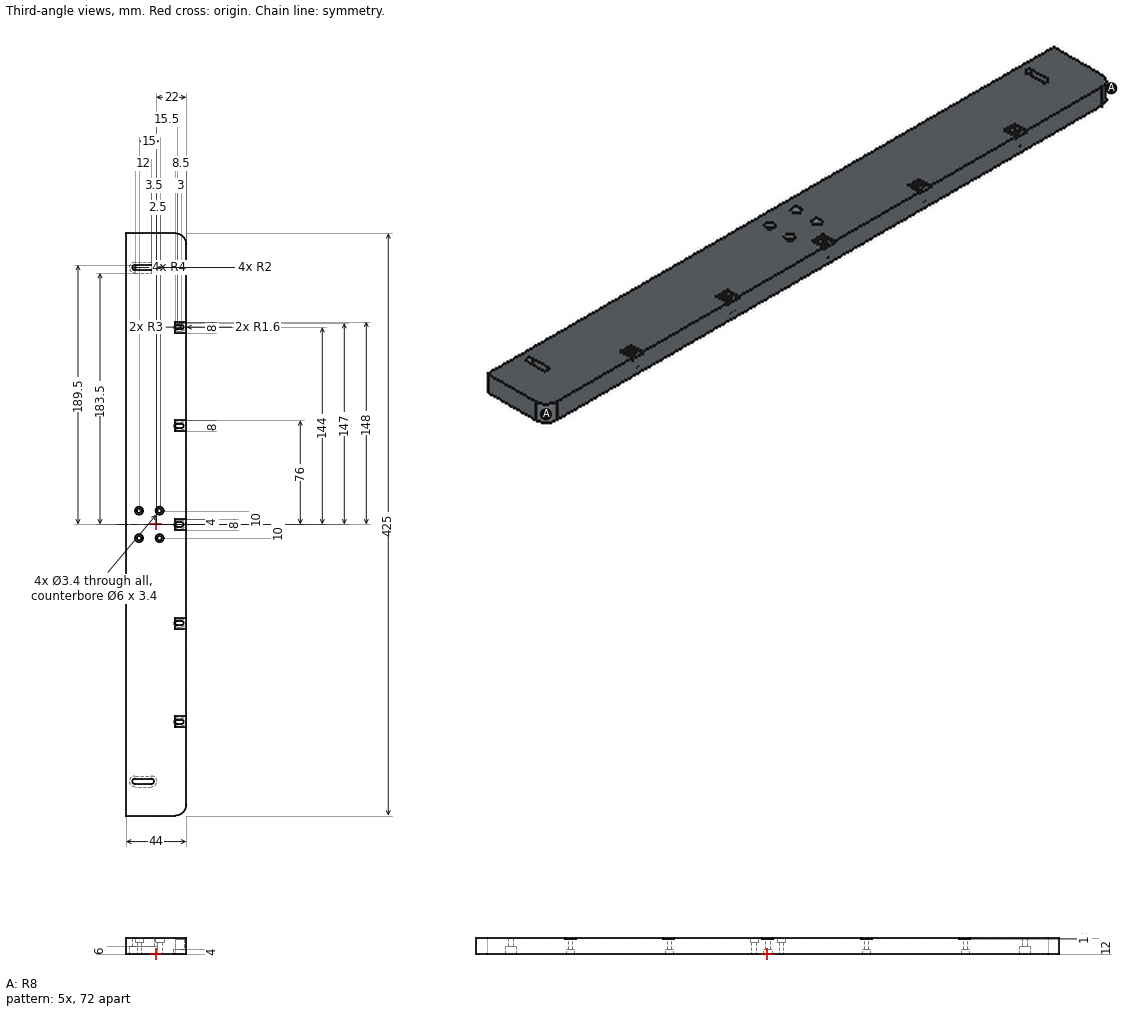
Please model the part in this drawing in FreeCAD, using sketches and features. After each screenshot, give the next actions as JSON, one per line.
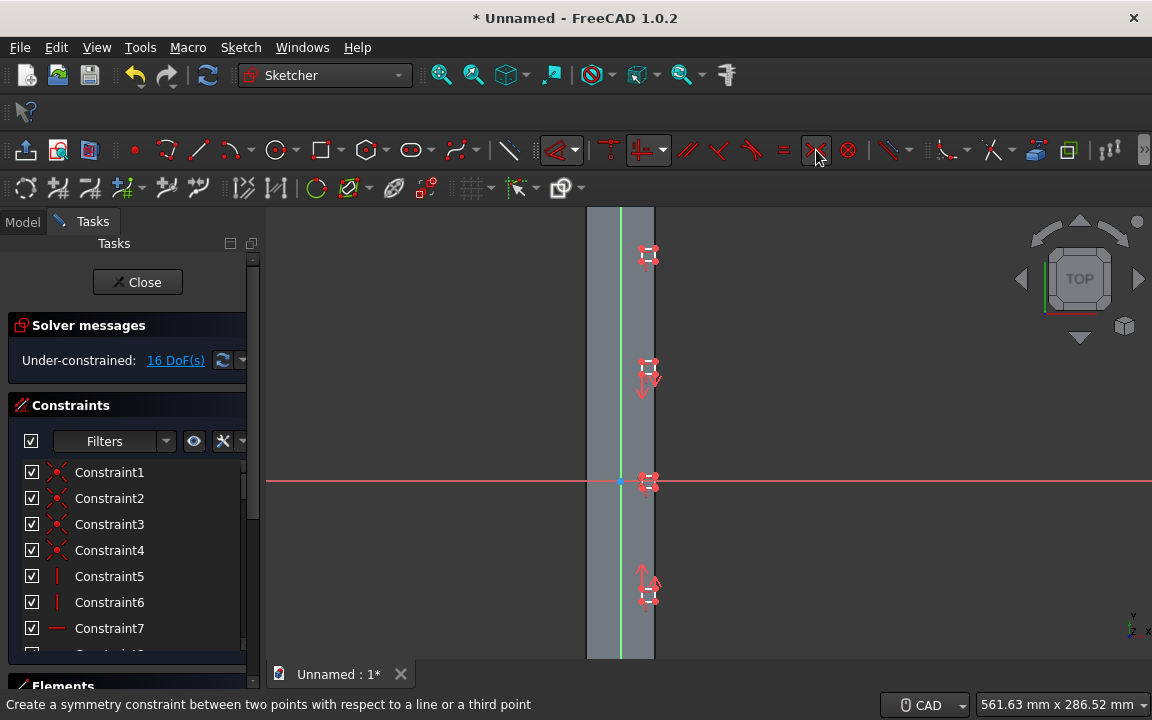
{"action": "left_click", "coordinate": [642, 261]}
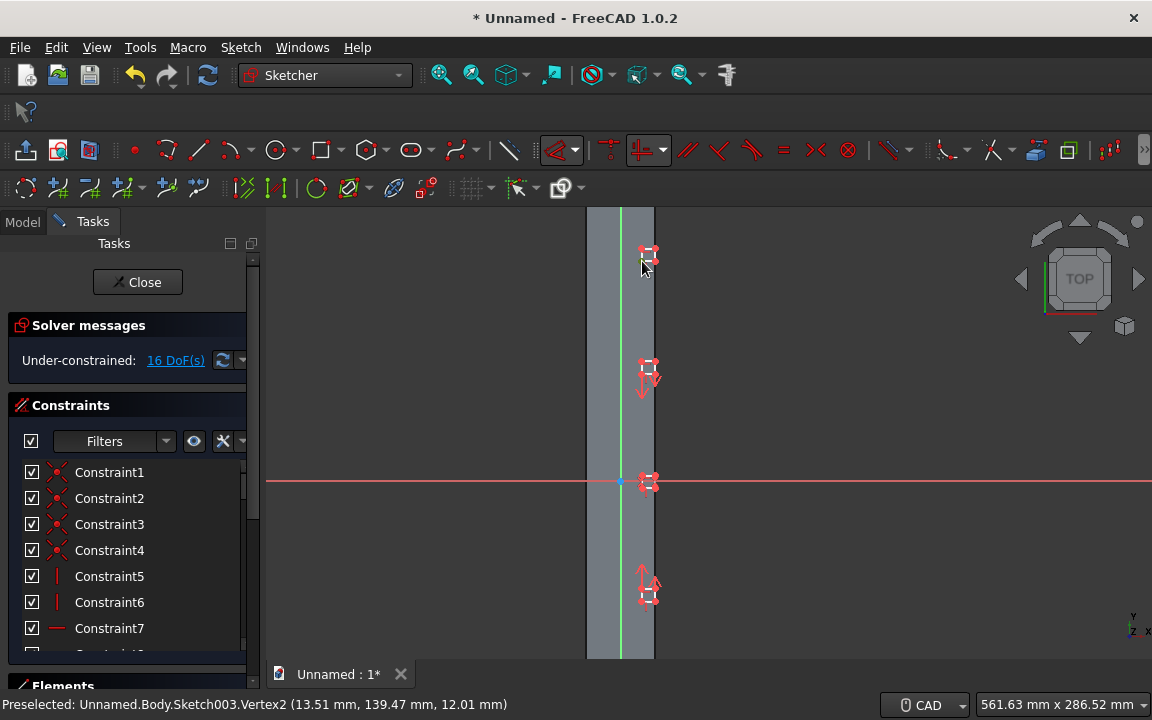
{"action": "scroll", "coordinate": [644, 374], "scroll_direction": "down", "scroll_amount": 3}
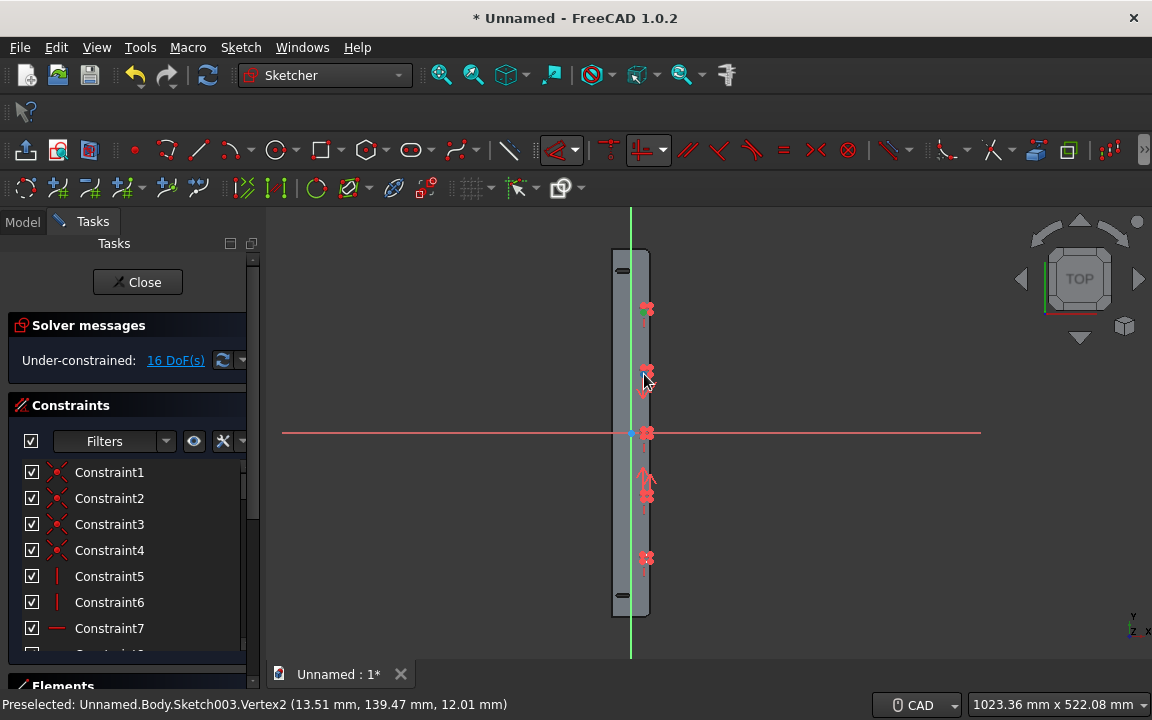
{"action": "scroll", "coordinate": [643, 555], "scroll_direction": "up", "scroll_amount": 3}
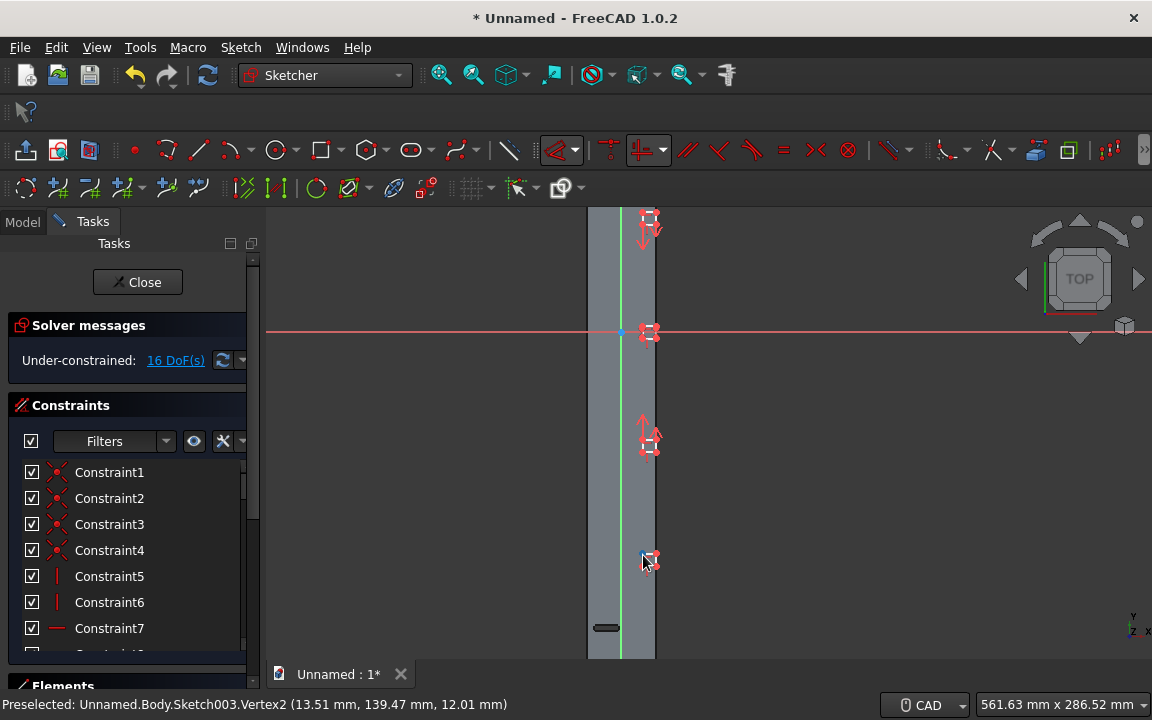
{"action": "left_click", "coordinate": [643, 554]}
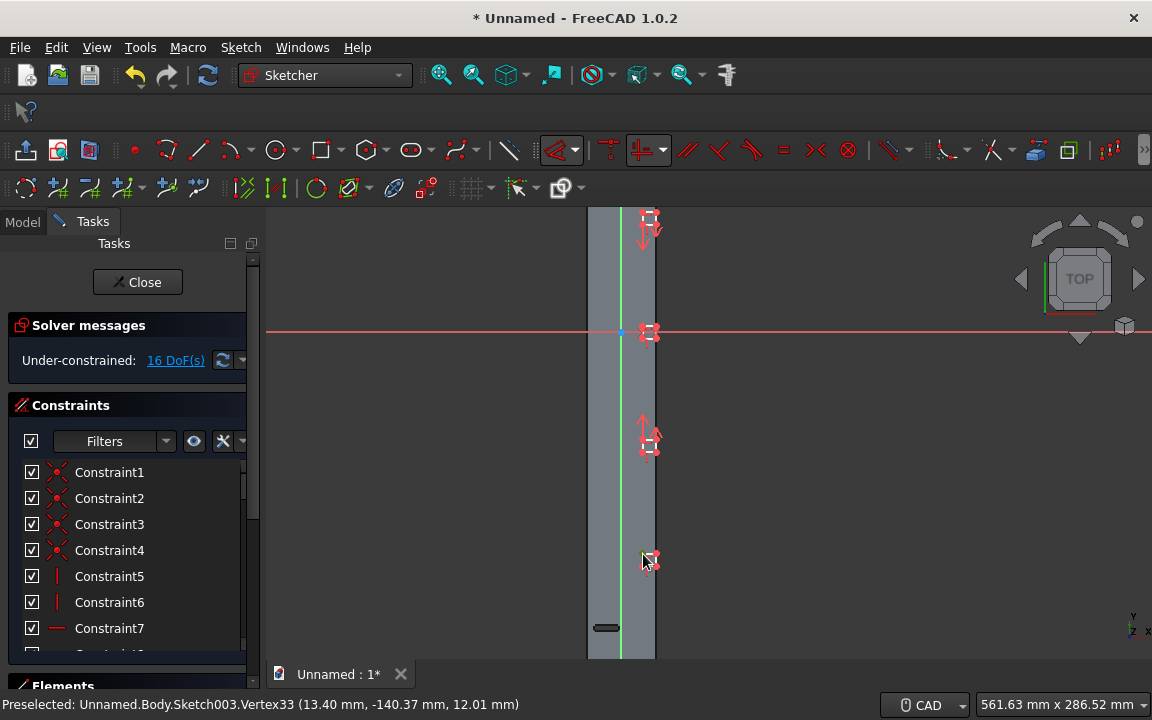
{"action": "left_click", "coordinate": [344, 332]}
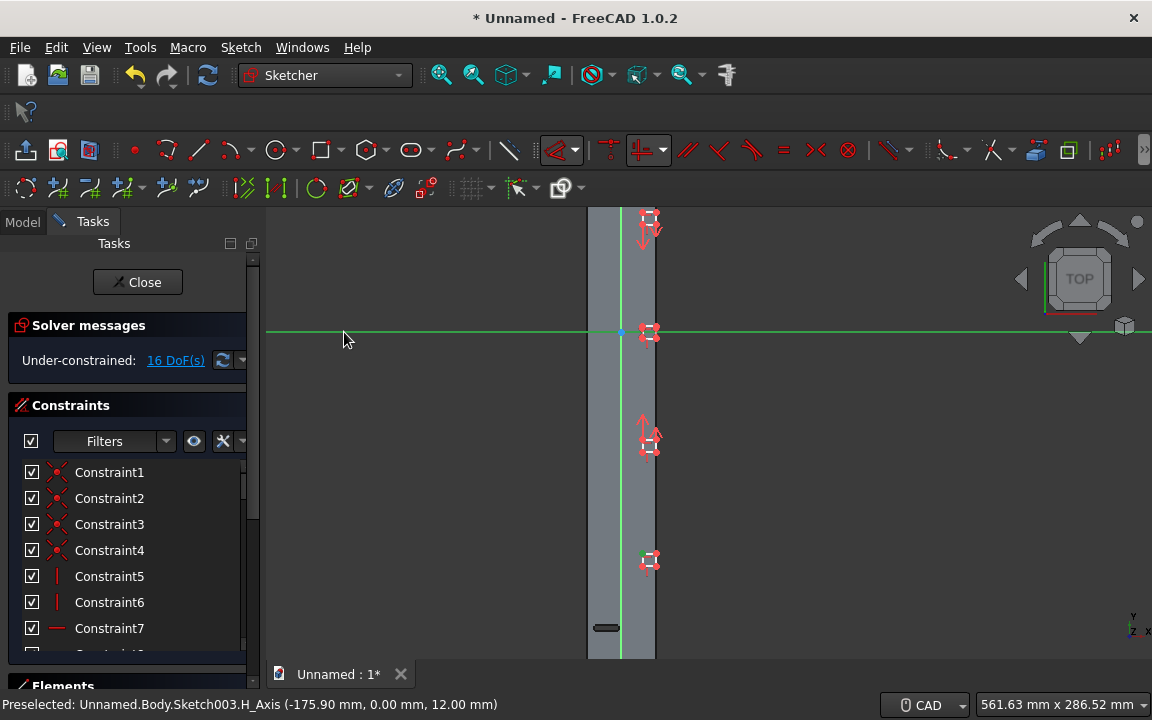
{"action": "key", "text": "s"}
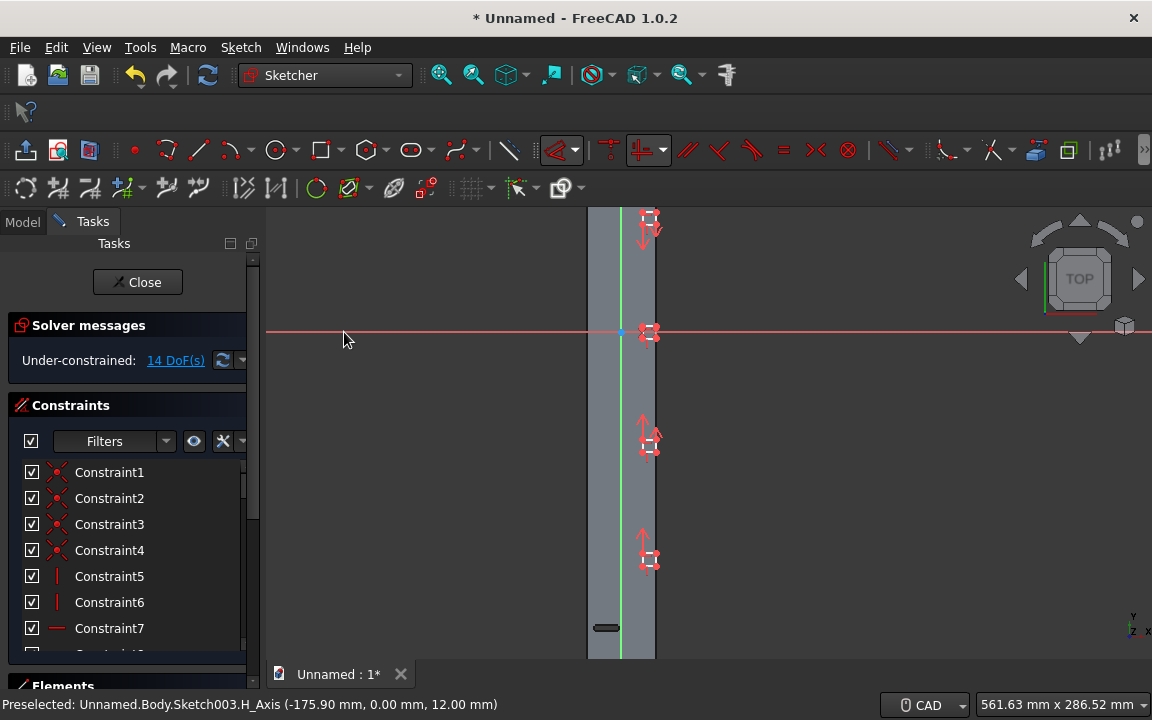
{"action": "scroll", "coordinate": [643, 555], "scroll_direction": "down", "scroll_amount": 3}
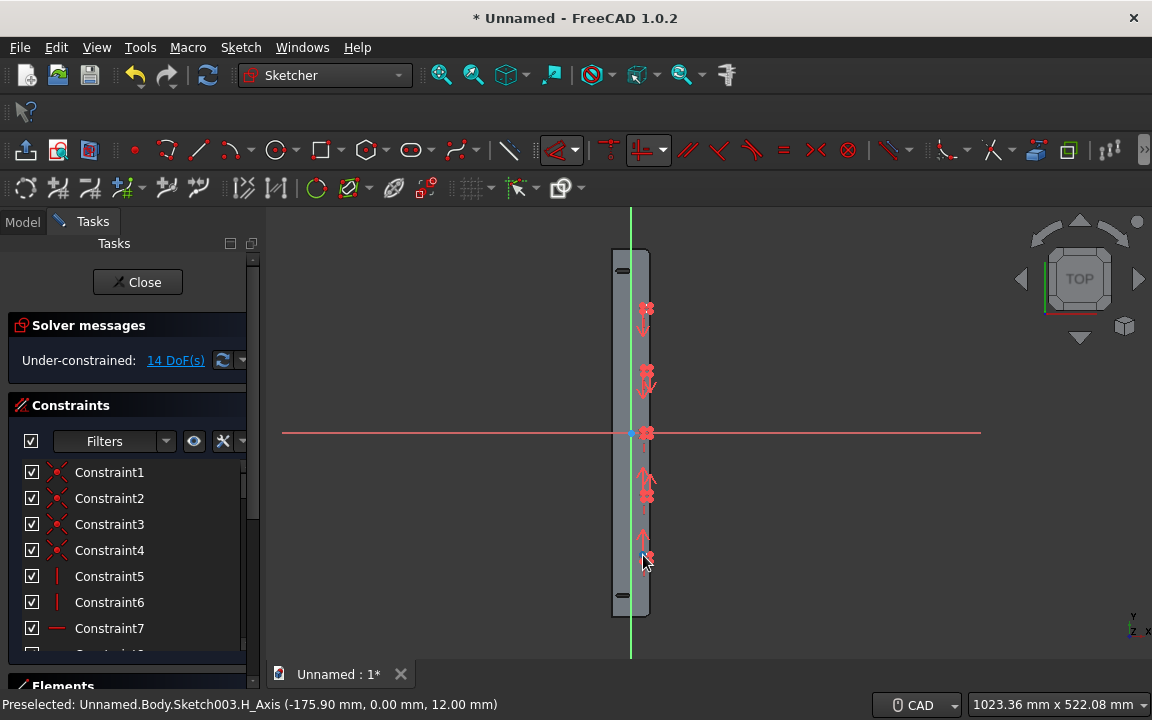
{"action": "scroll", "coordinate": [650, 305], "scroll_direction": "up", "scroll_amount": 4}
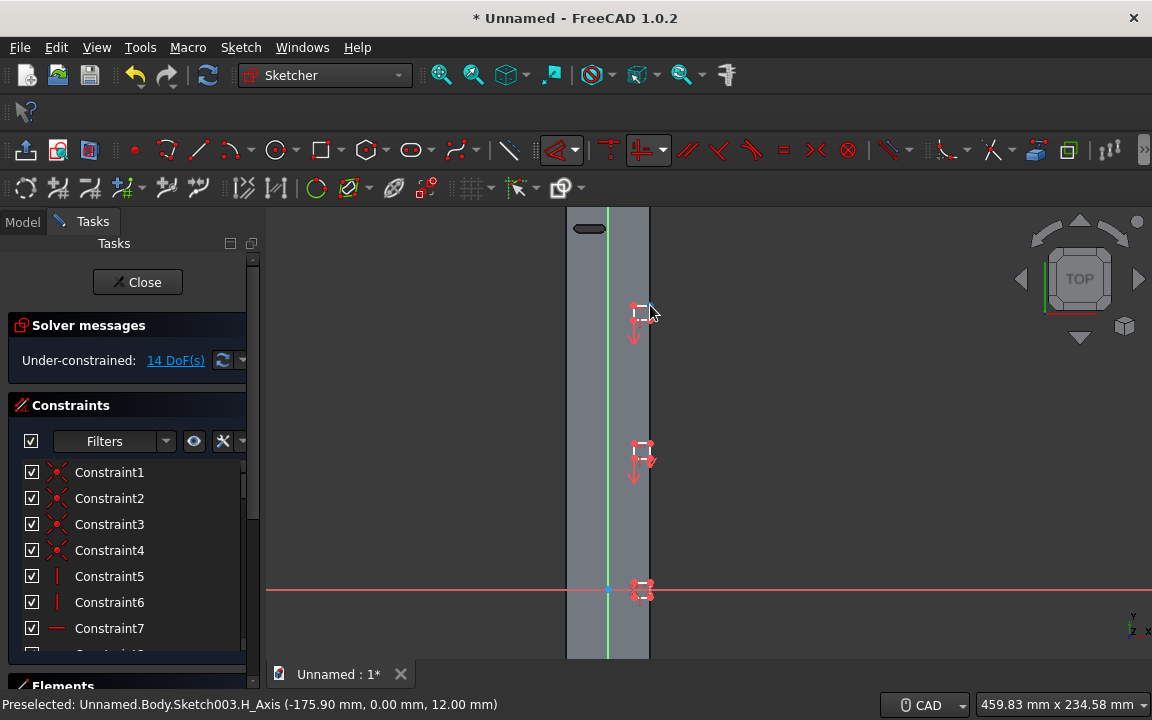
{"action": "left_click", "coordinate": [650, 306]}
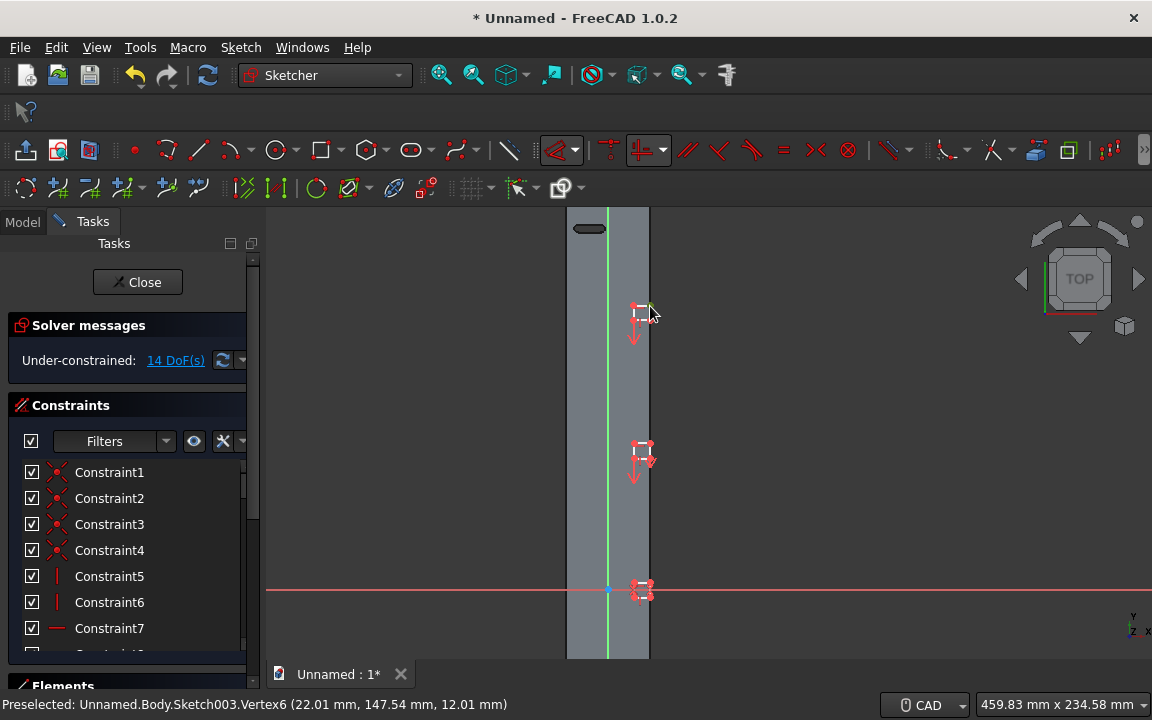
{"action": "scroll", "coordinate": [650, 305], "scroll_direction": "down", "scroll_amount": 4}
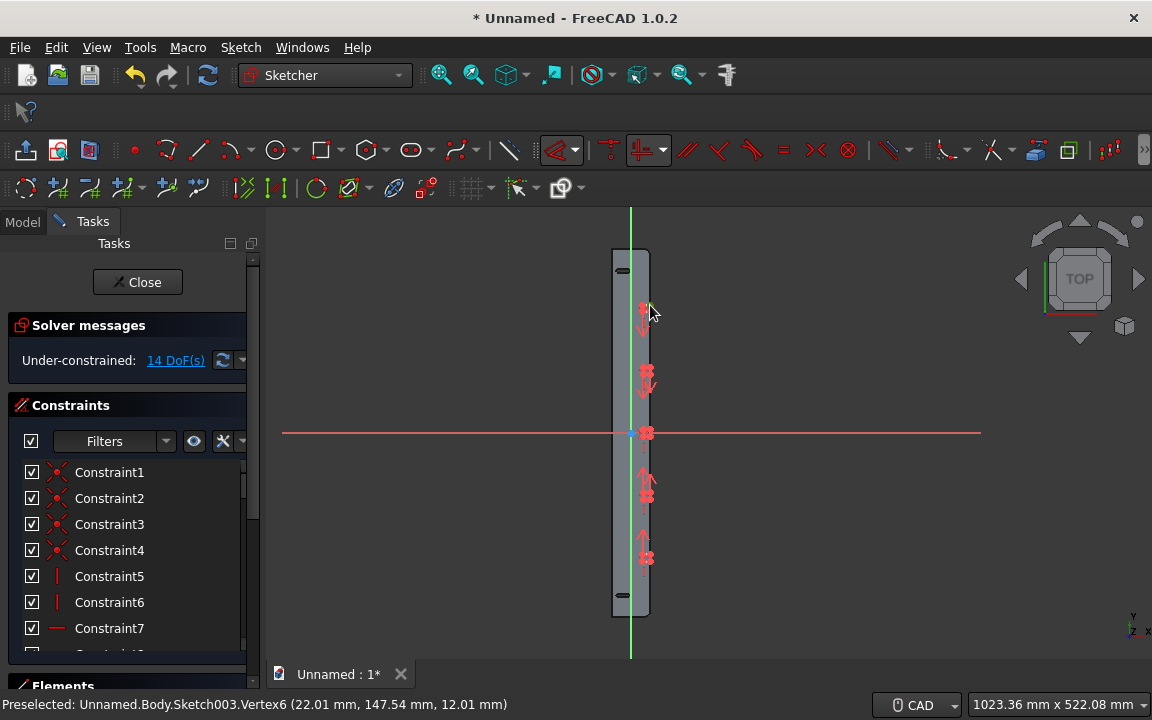
{"action": "scroll", "coordinate": [650, 562], "scroll_direction": "up", "scroll_amount": 3}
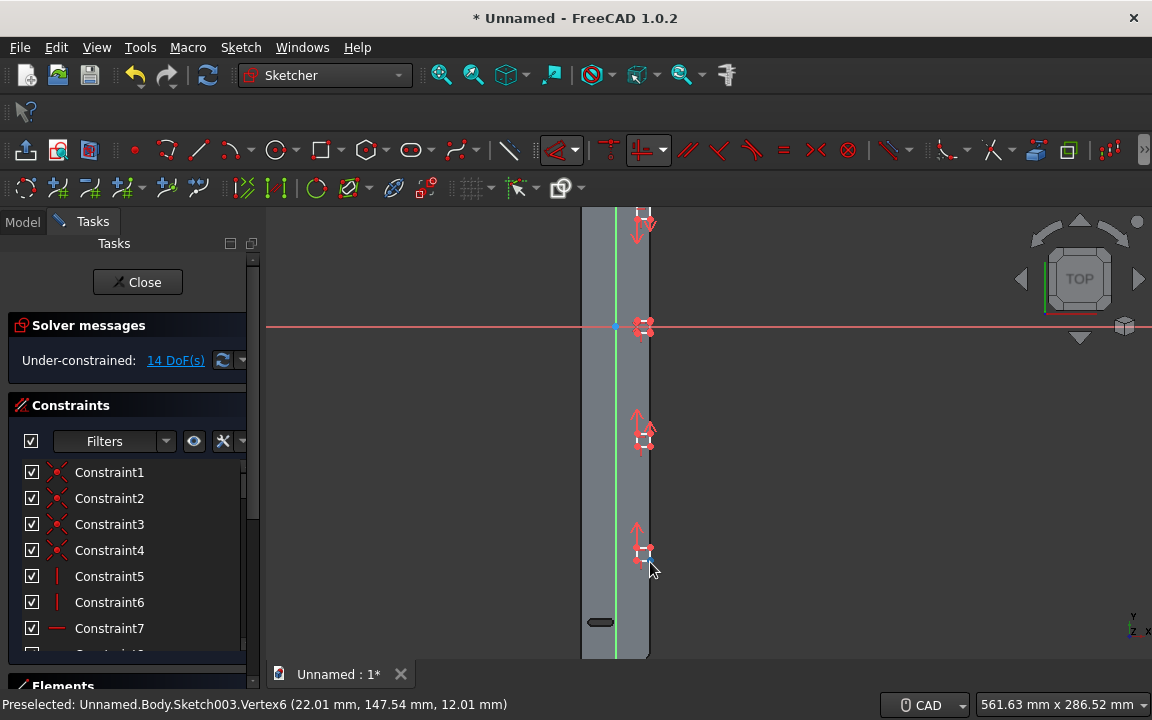
{"action": "left_click", "coordinate": [650, 561]}